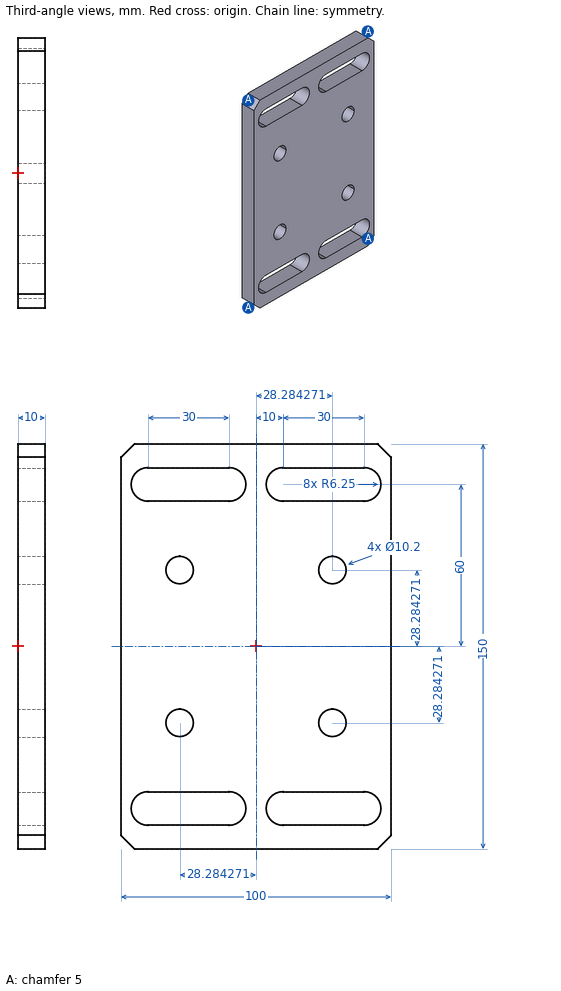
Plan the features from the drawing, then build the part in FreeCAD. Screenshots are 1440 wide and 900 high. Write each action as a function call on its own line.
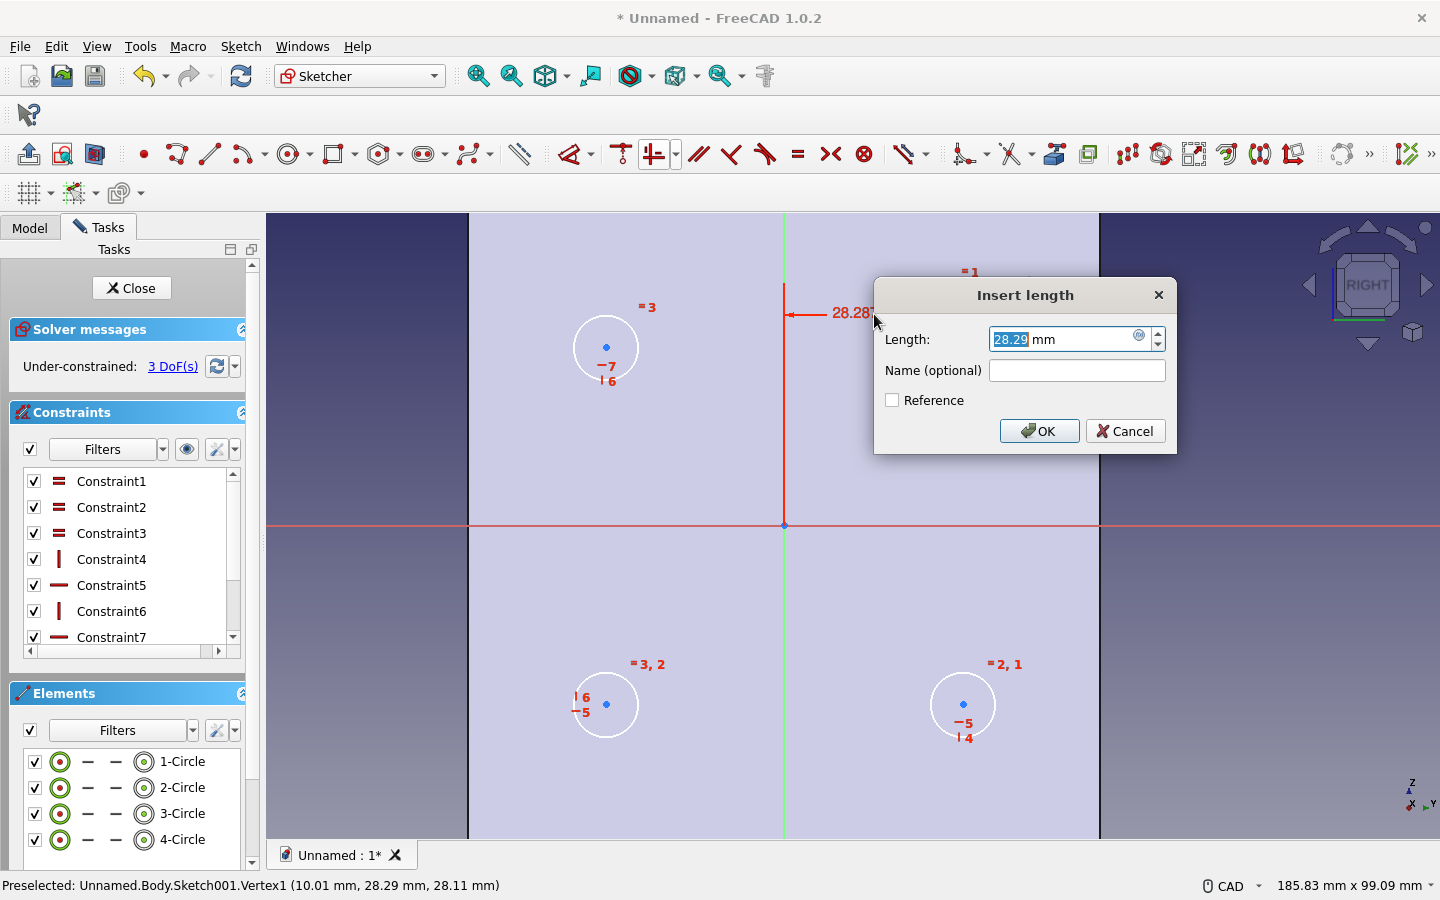
text(28.284271)
key(Return)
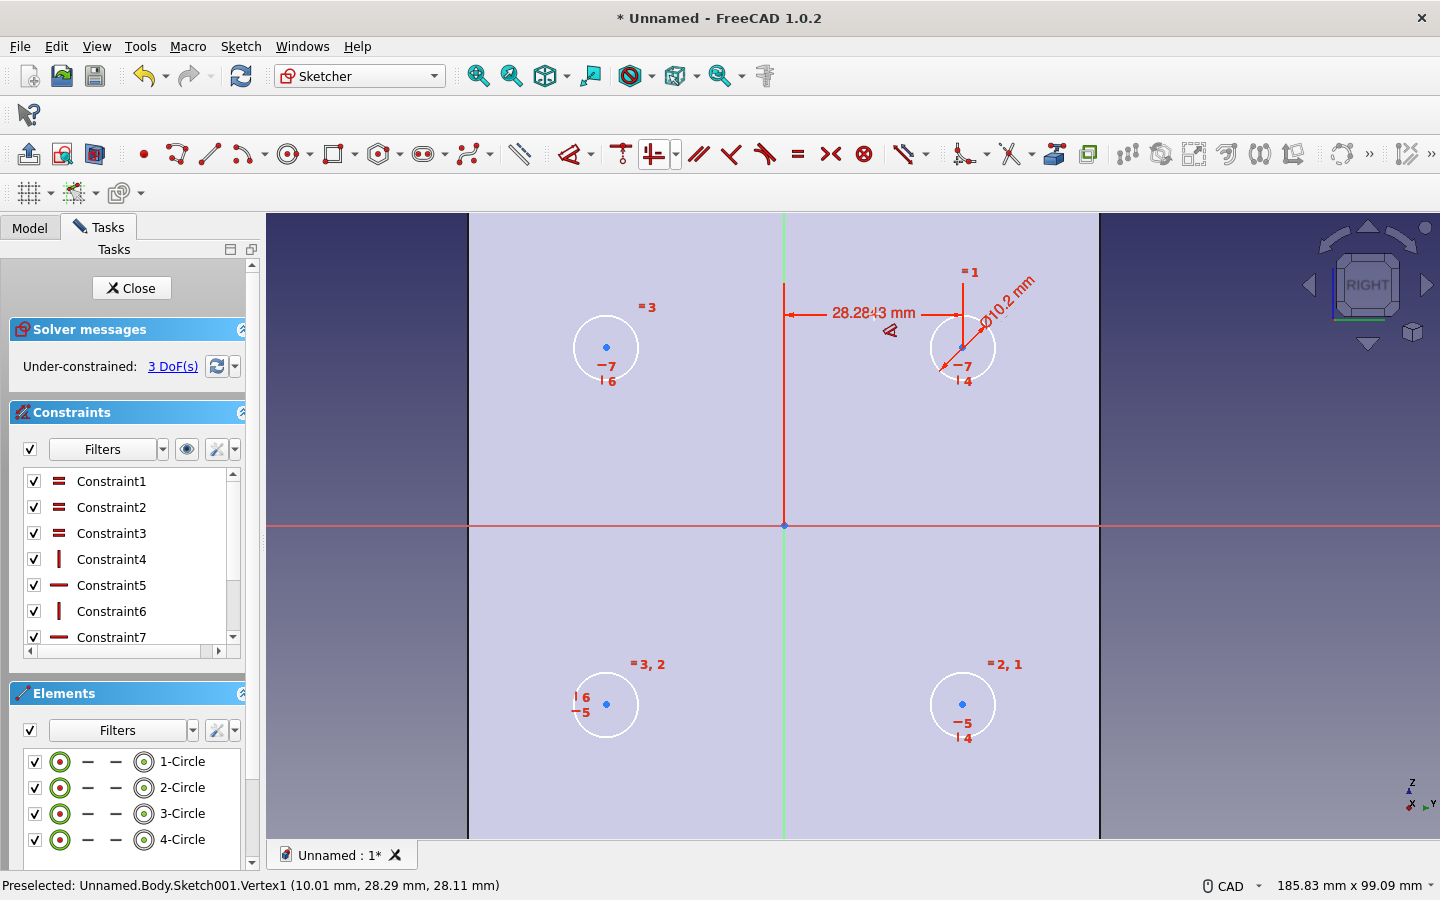
click(963, 348)
click(997, 437)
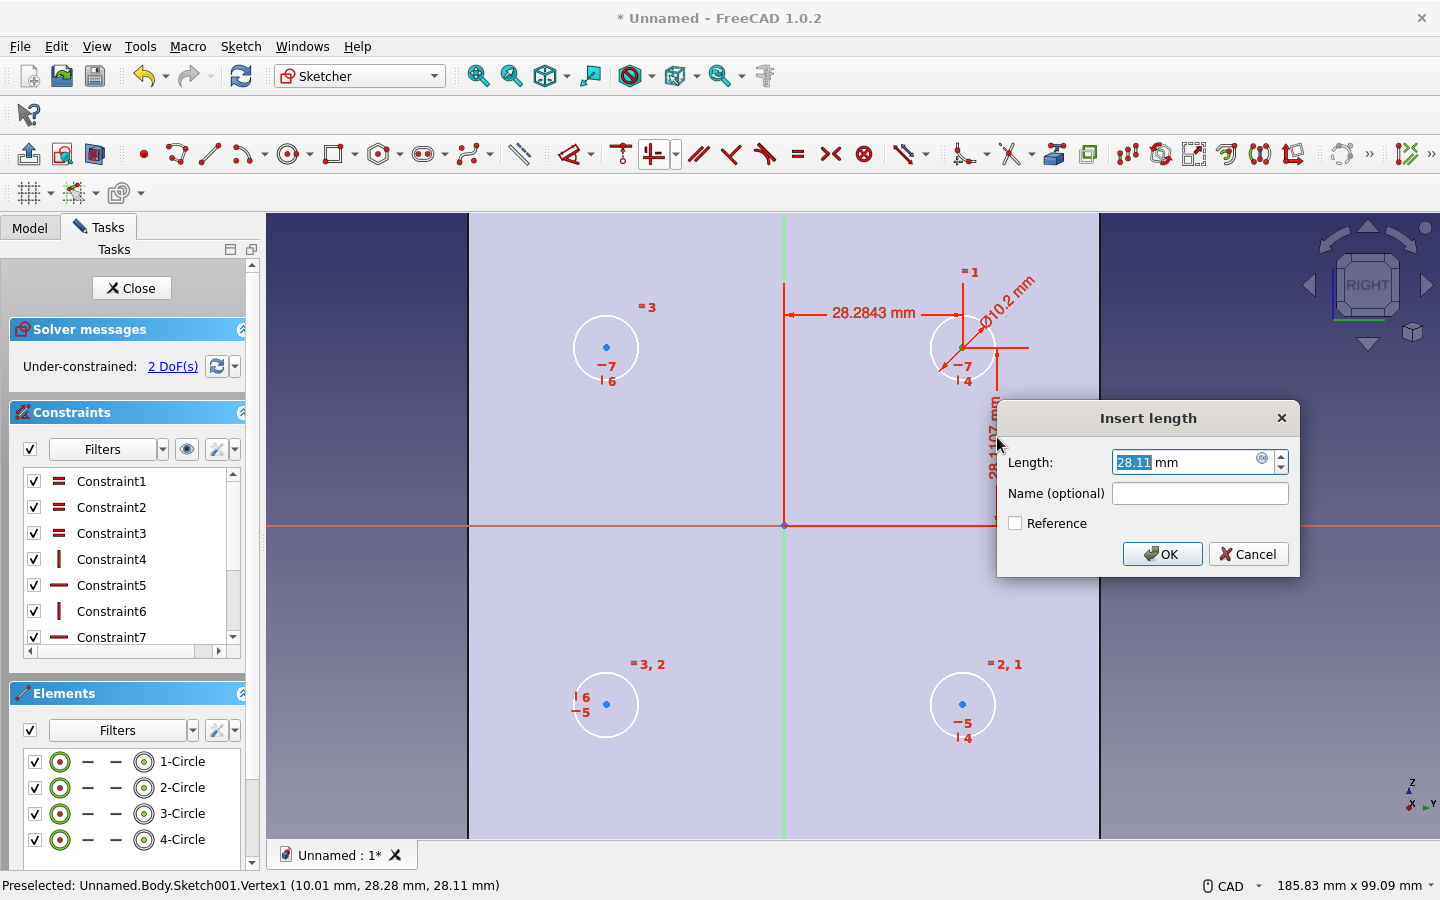
text(28.284271)
key(Return)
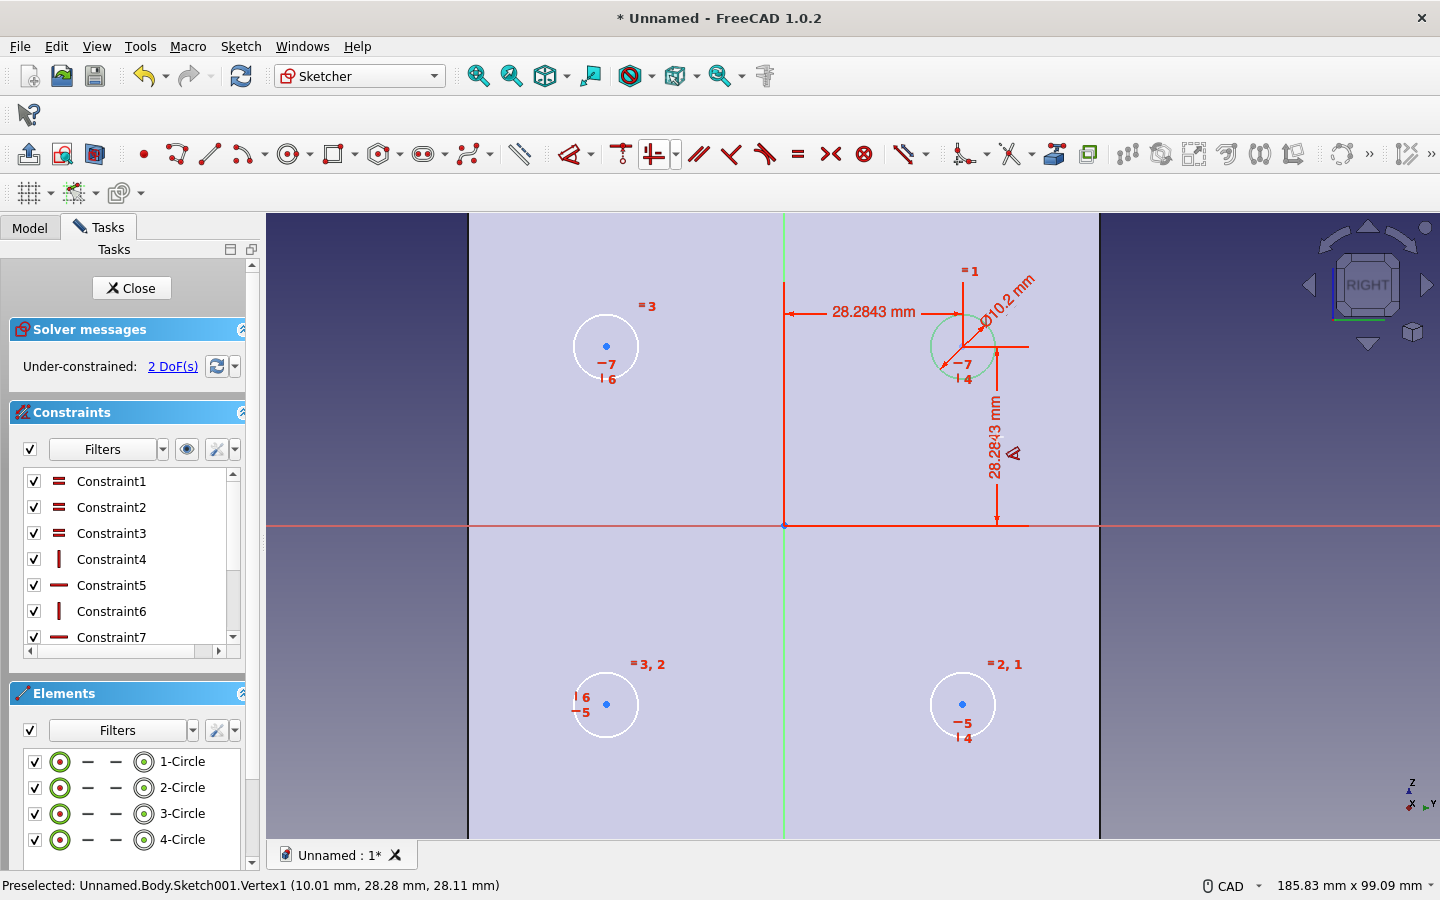
click(963, 705)
click(997, 615)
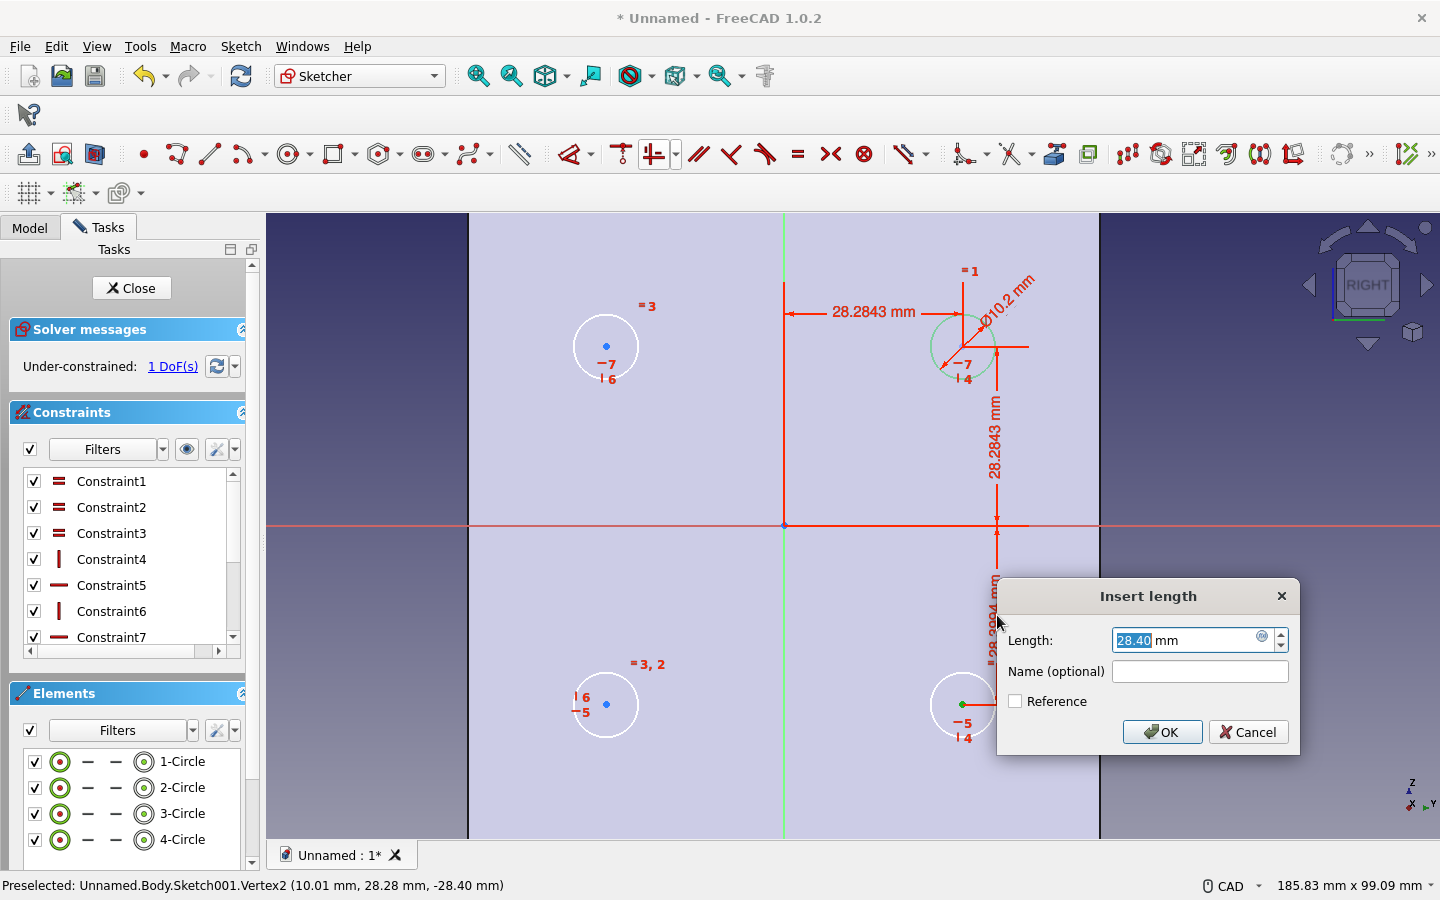
text(28.284271)
key(Return)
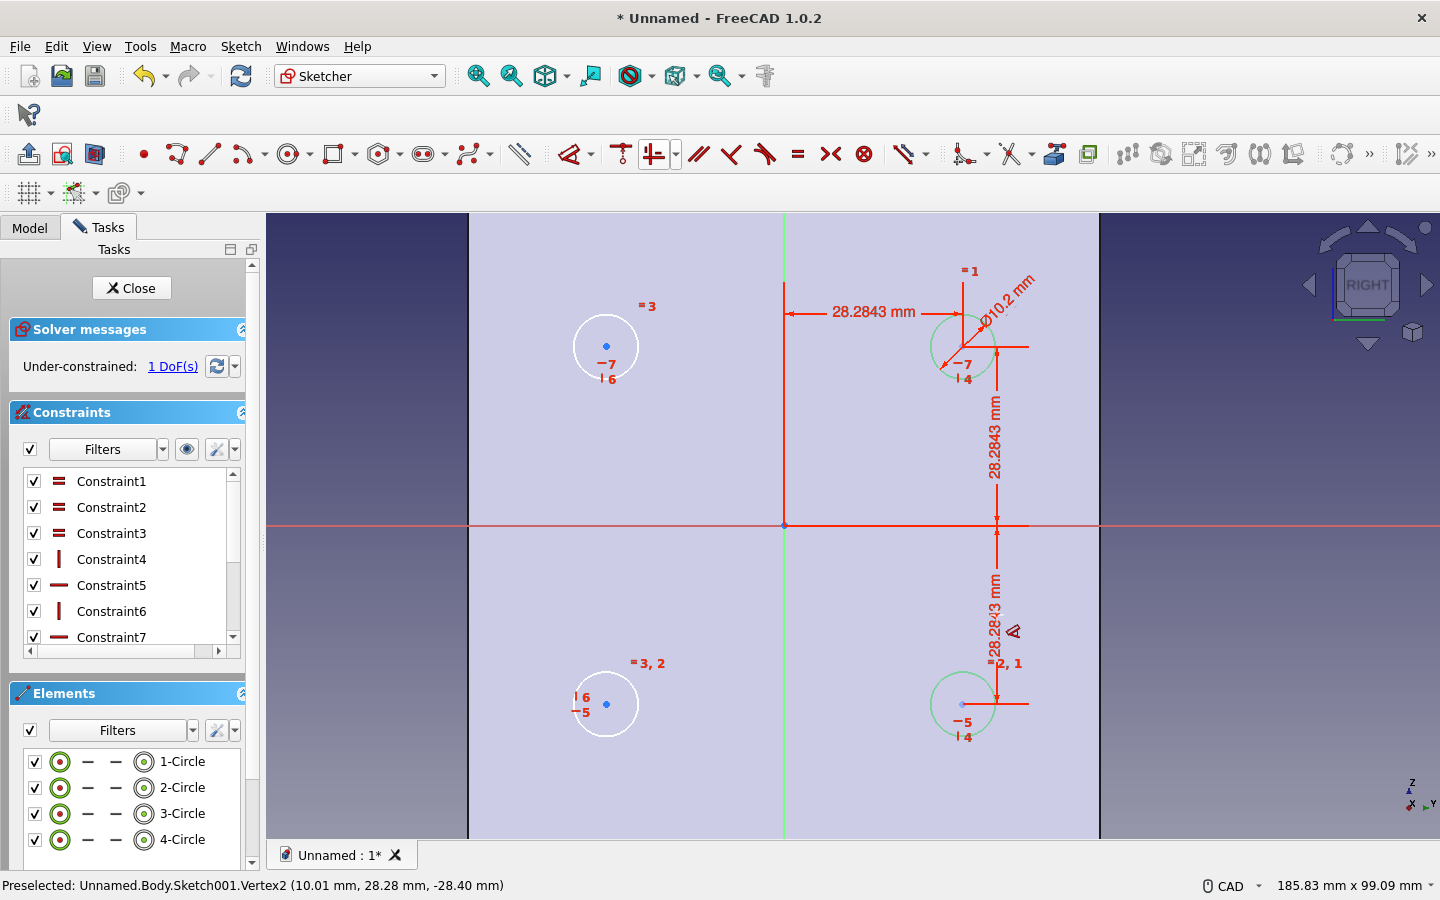
click(606, 704)
click(695, 738)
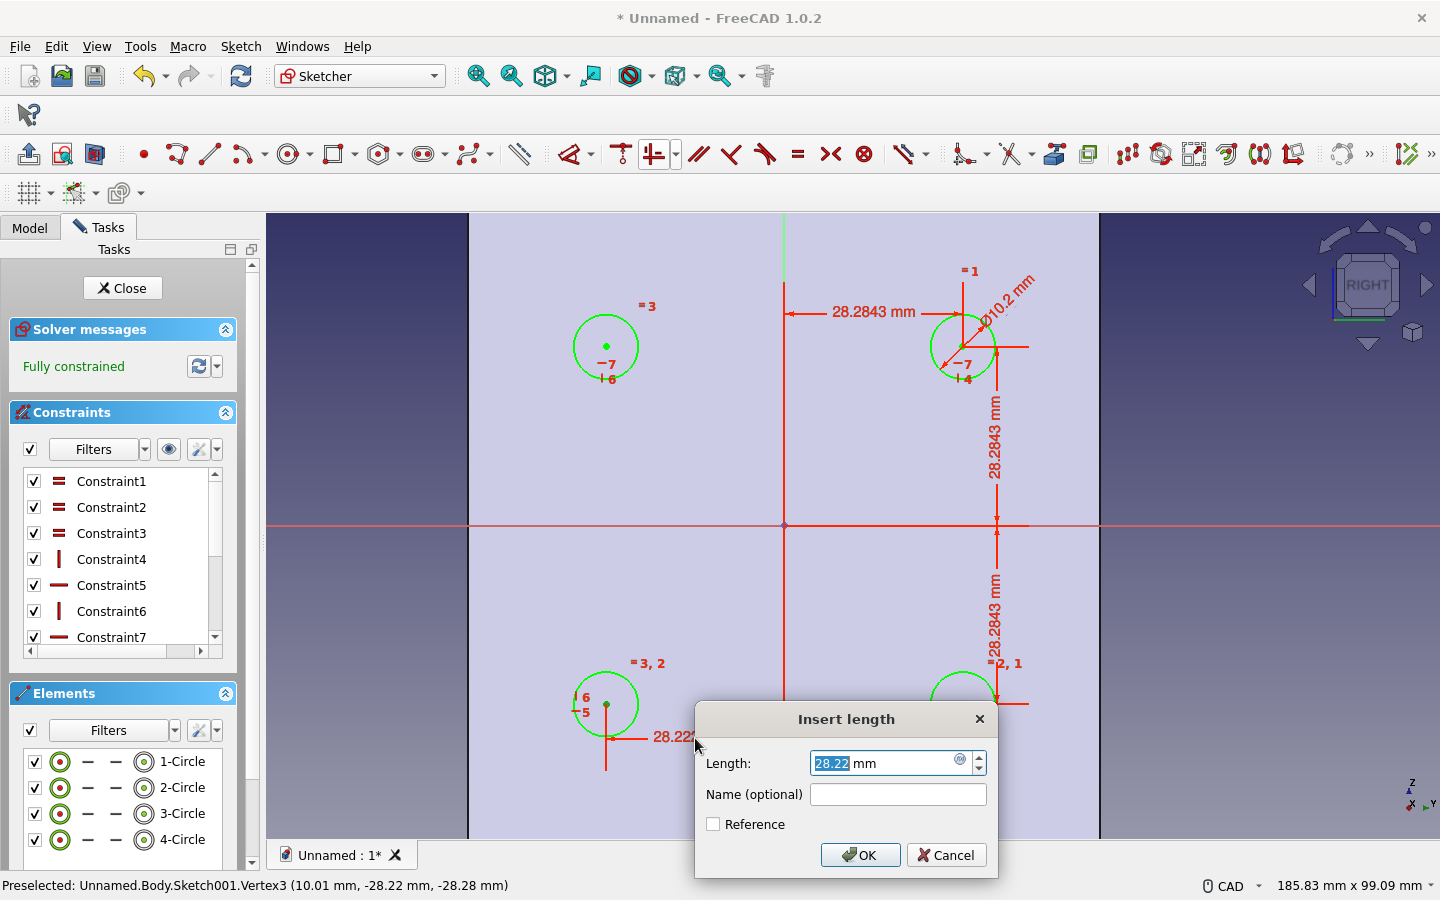
text(28.284271)
key(Return)
key(Escape)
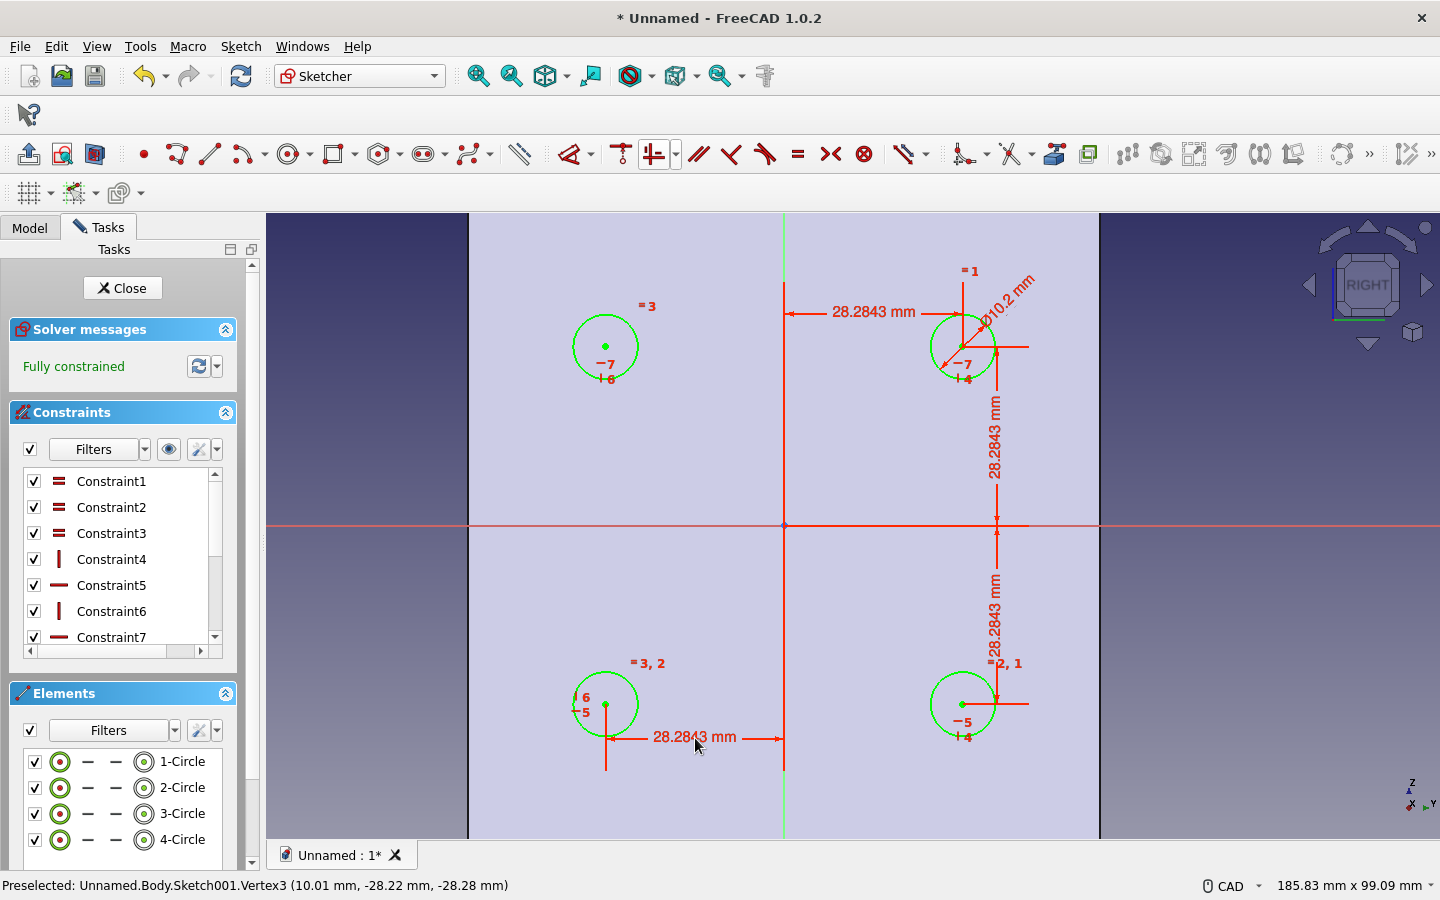
click(123, 288)